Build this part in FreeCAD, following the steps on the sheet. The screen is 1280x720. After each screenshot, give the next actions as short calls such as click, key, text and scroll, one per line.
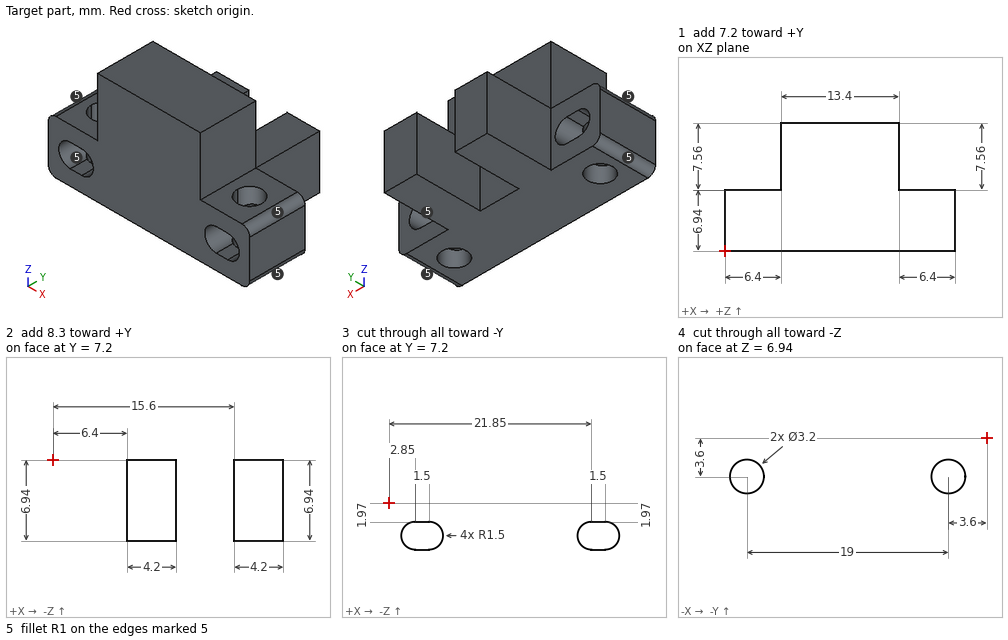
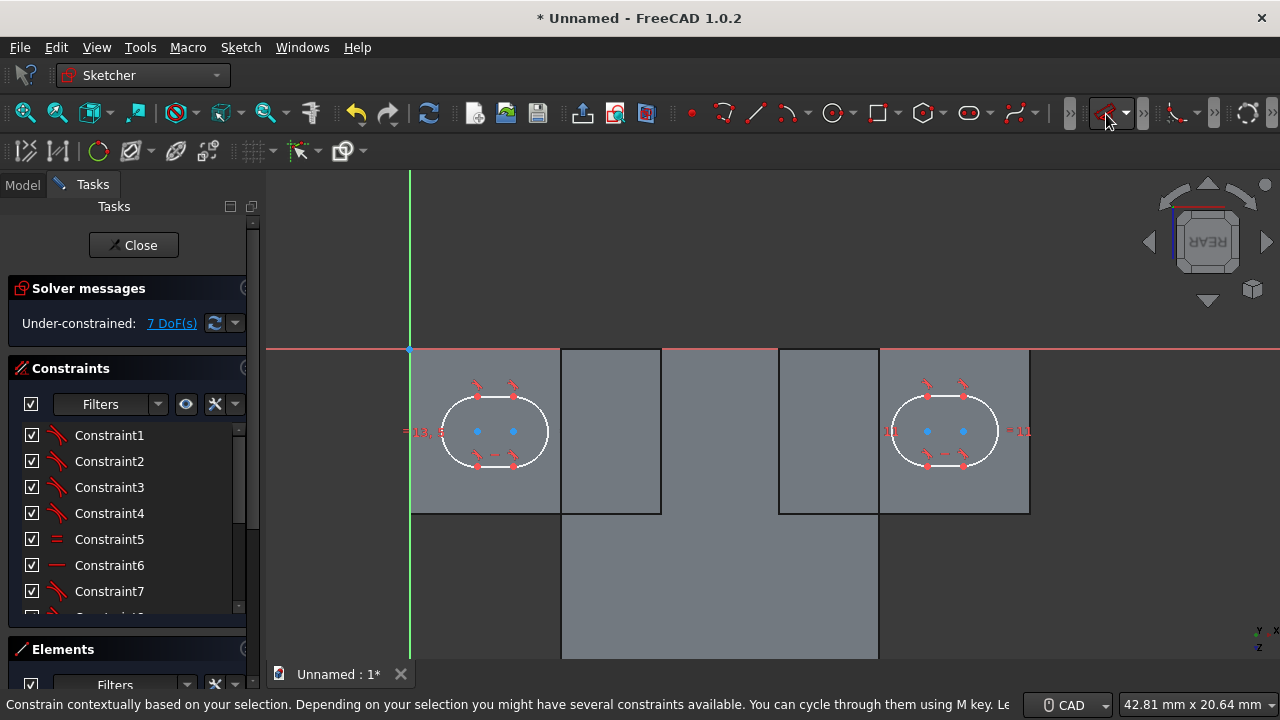
click(449, 411)
click(423, 392)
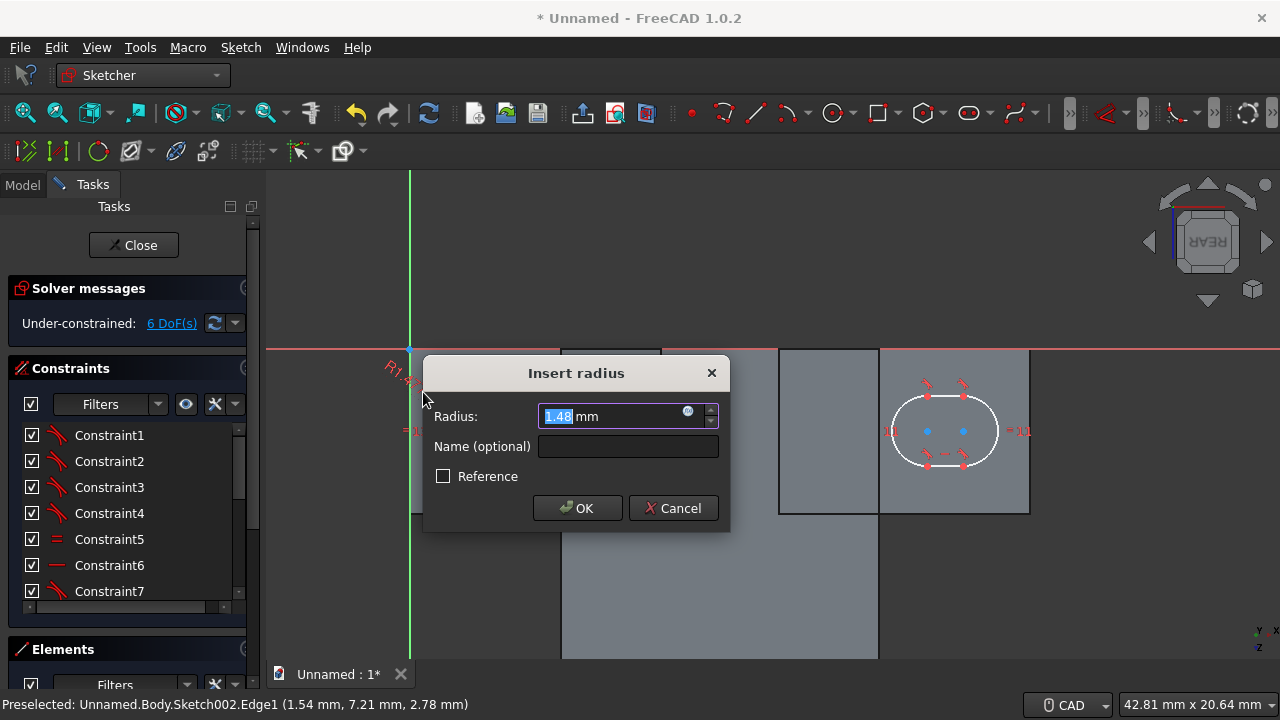
text(1.5)
key(Return)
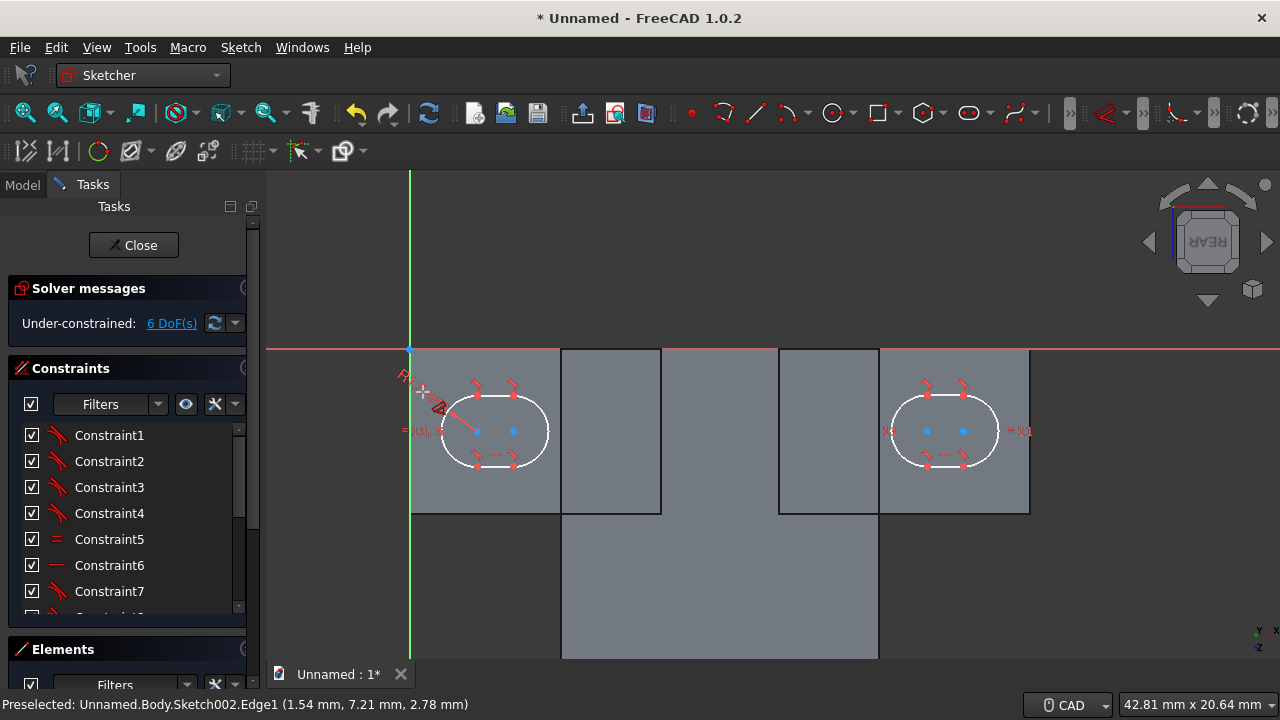
scroll(488, 396, up, 2)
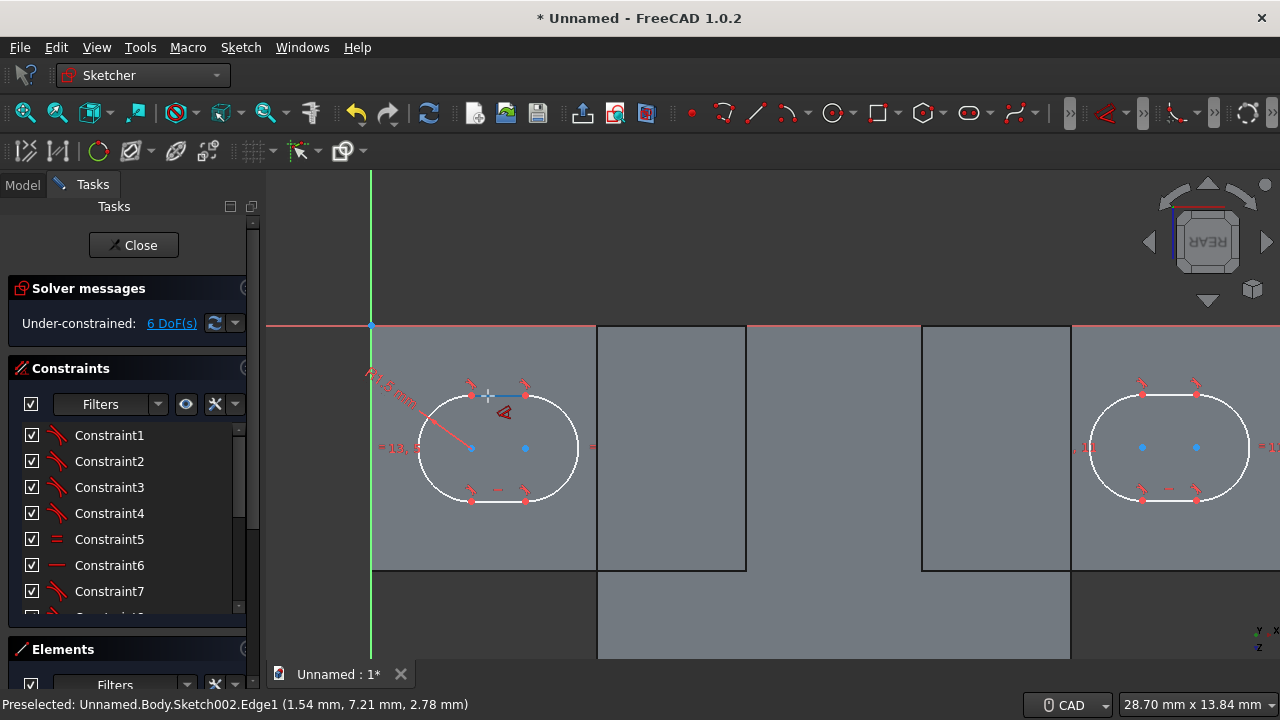
click(488, 396)
click(498, 362)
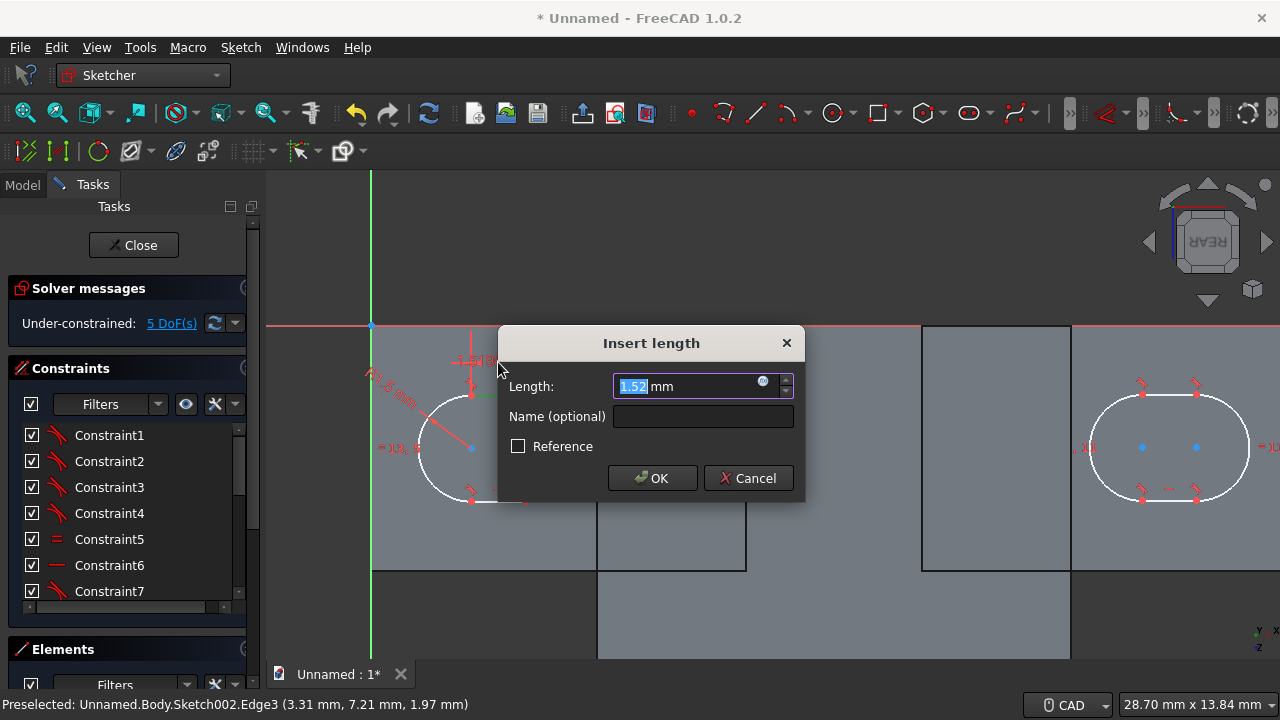
text(1.5)
key(Return)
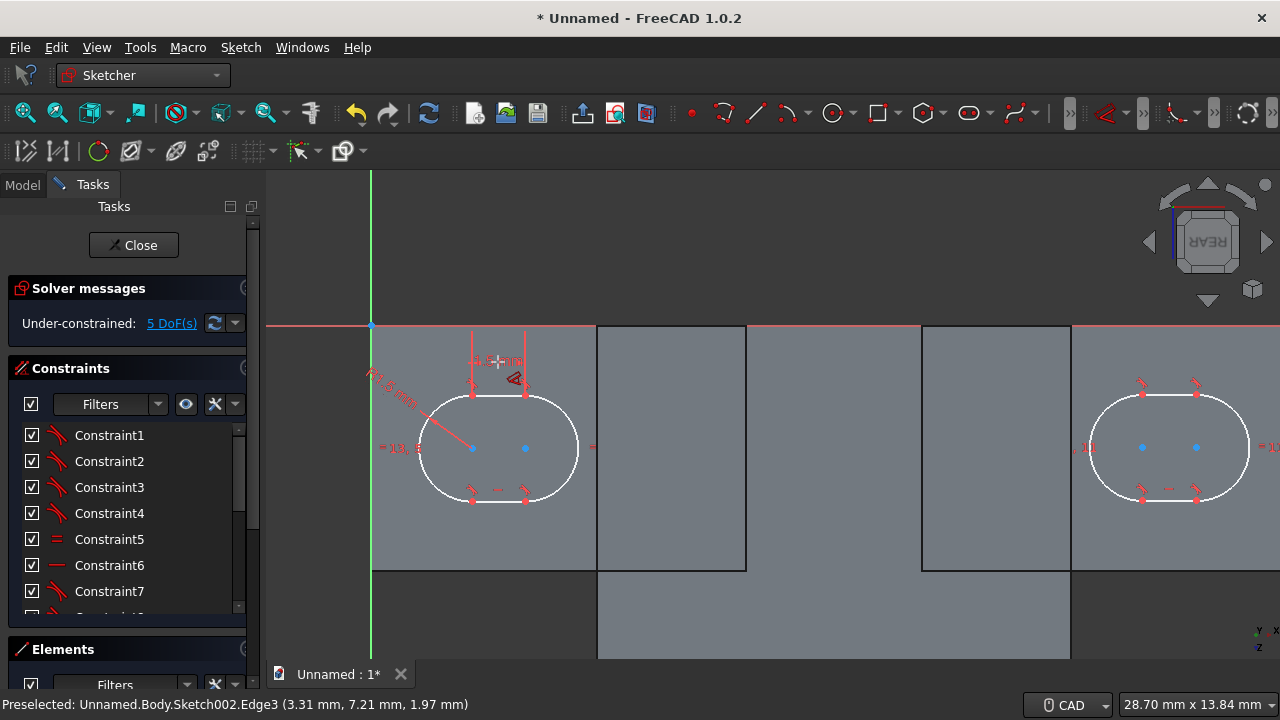
scroll(489, 416, down, 2)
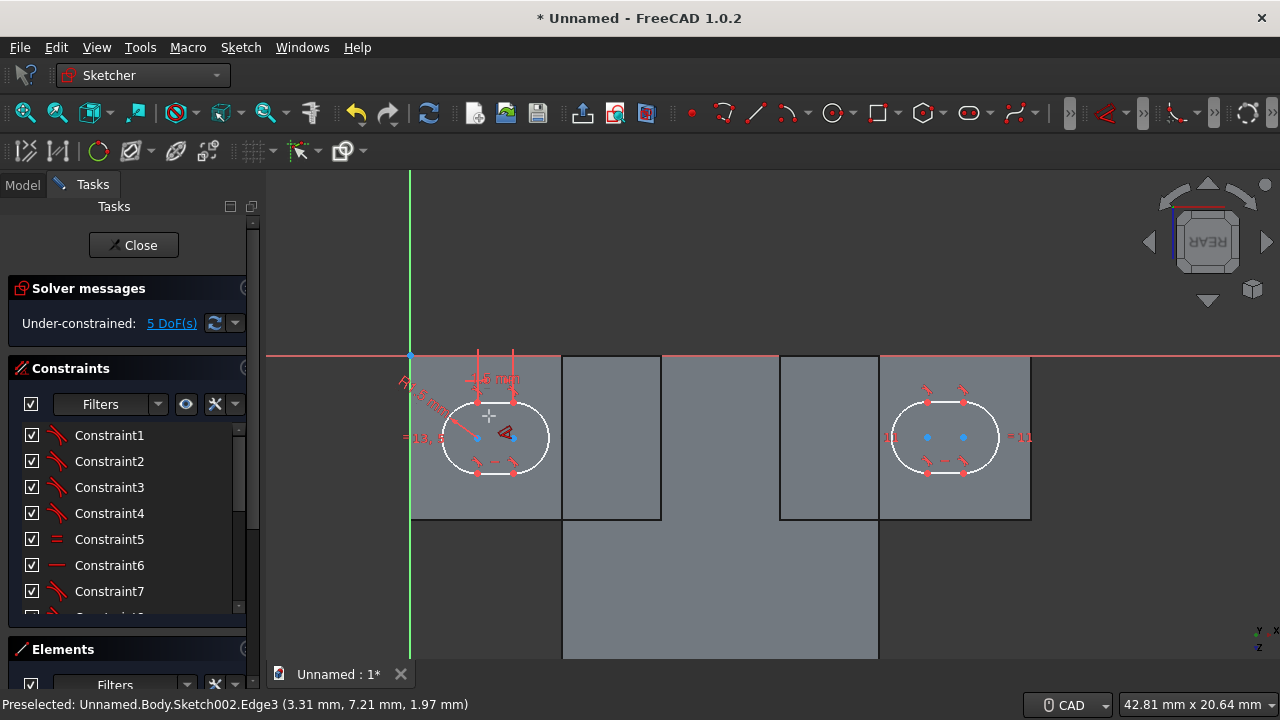
scroll(938, 402, up, 2)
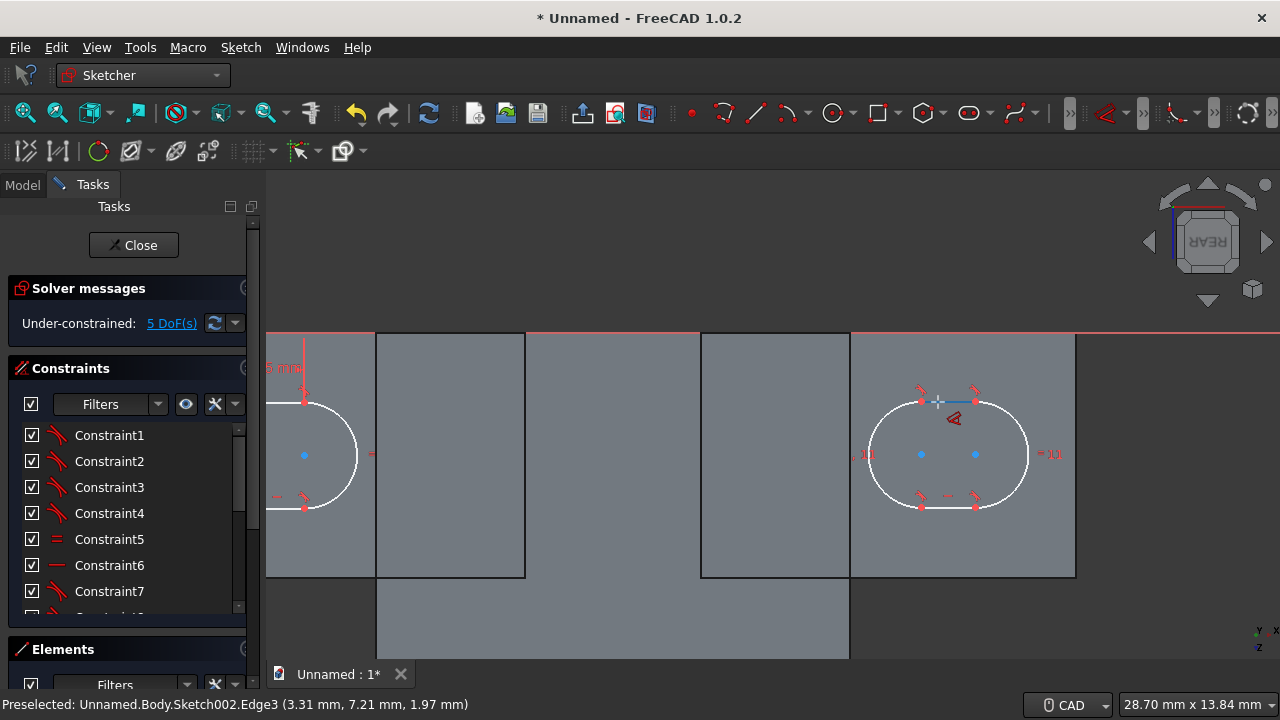
click(938, 402)
click(949, 368)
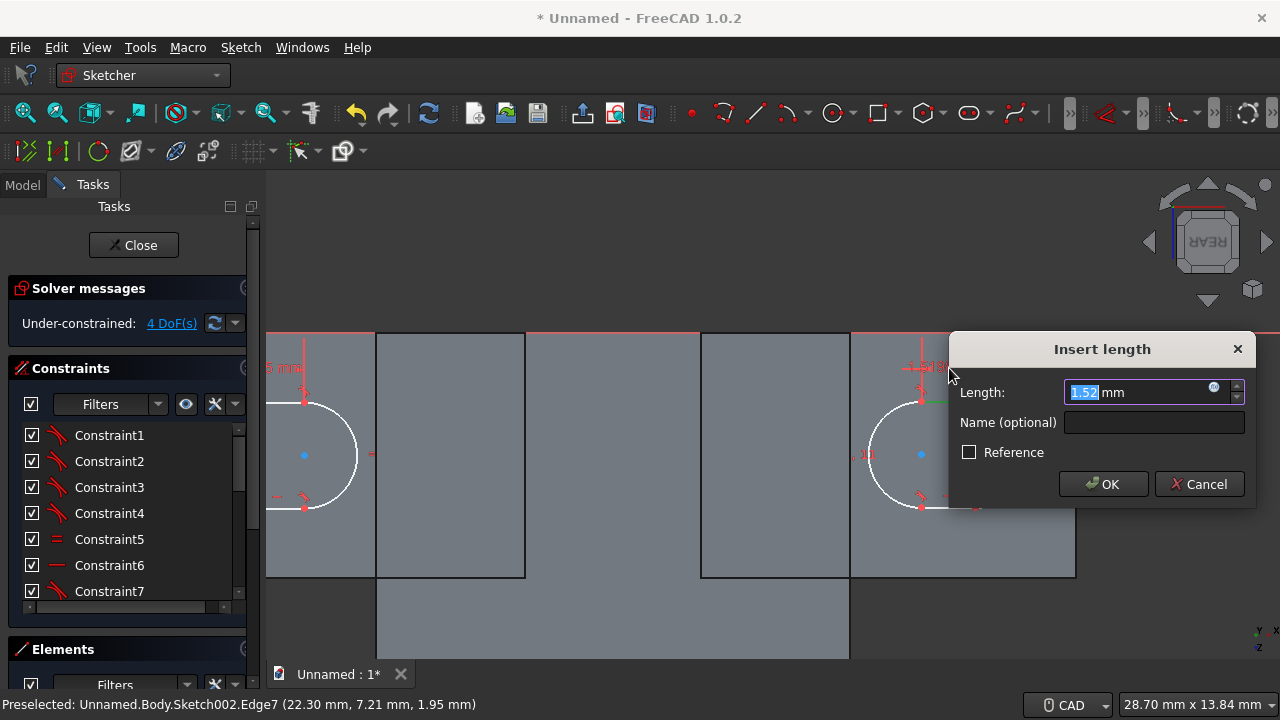
text(1.5)
key(Return)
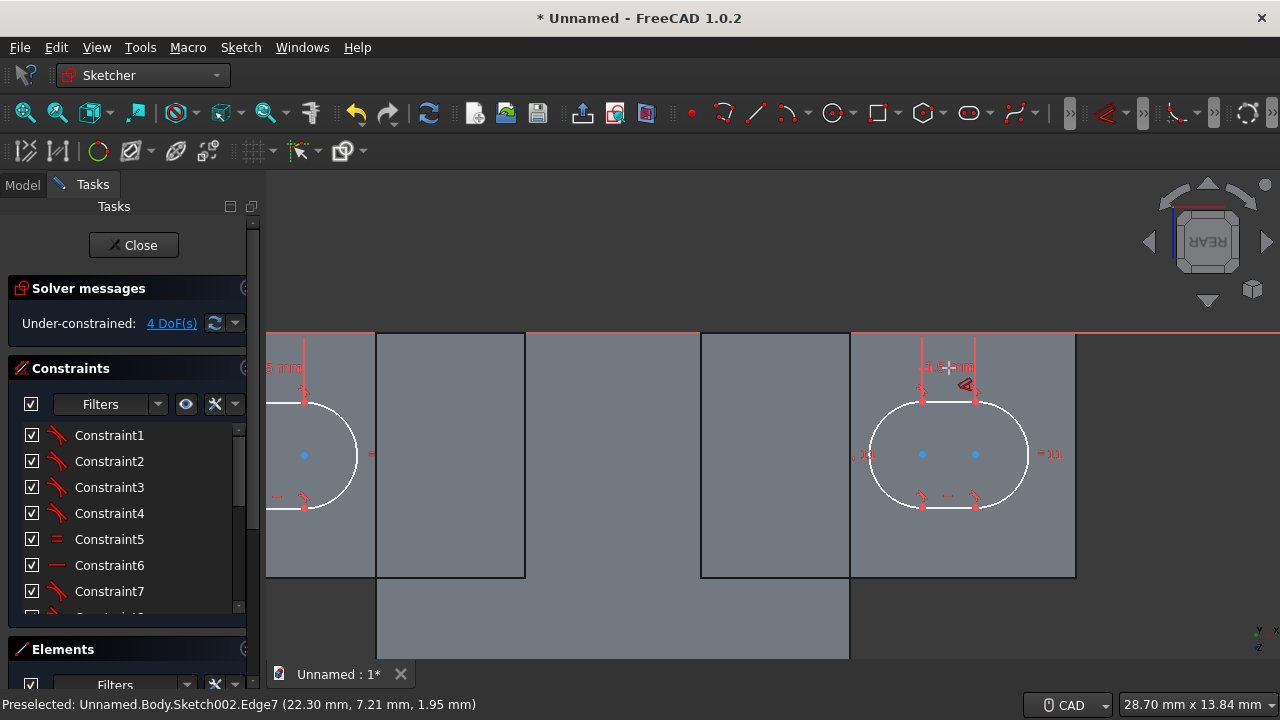
scroll(939, 402, down, 2)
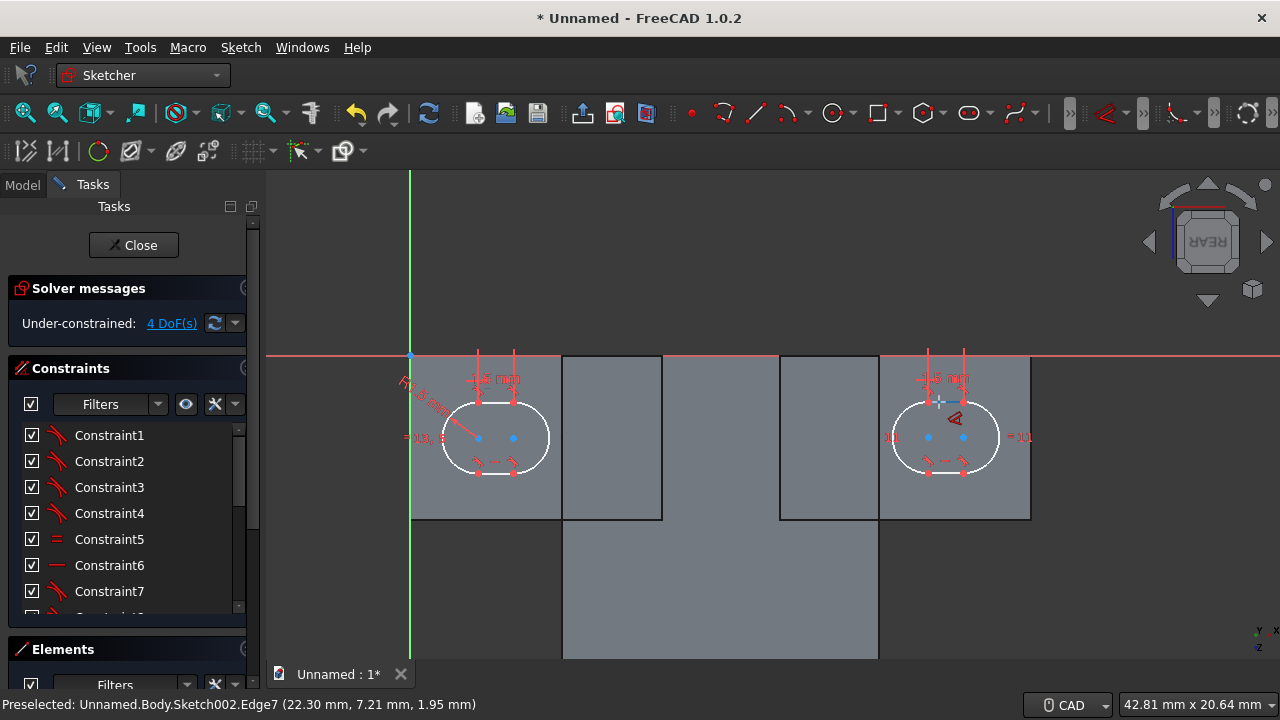
click(478, 403)
click(444, 322)